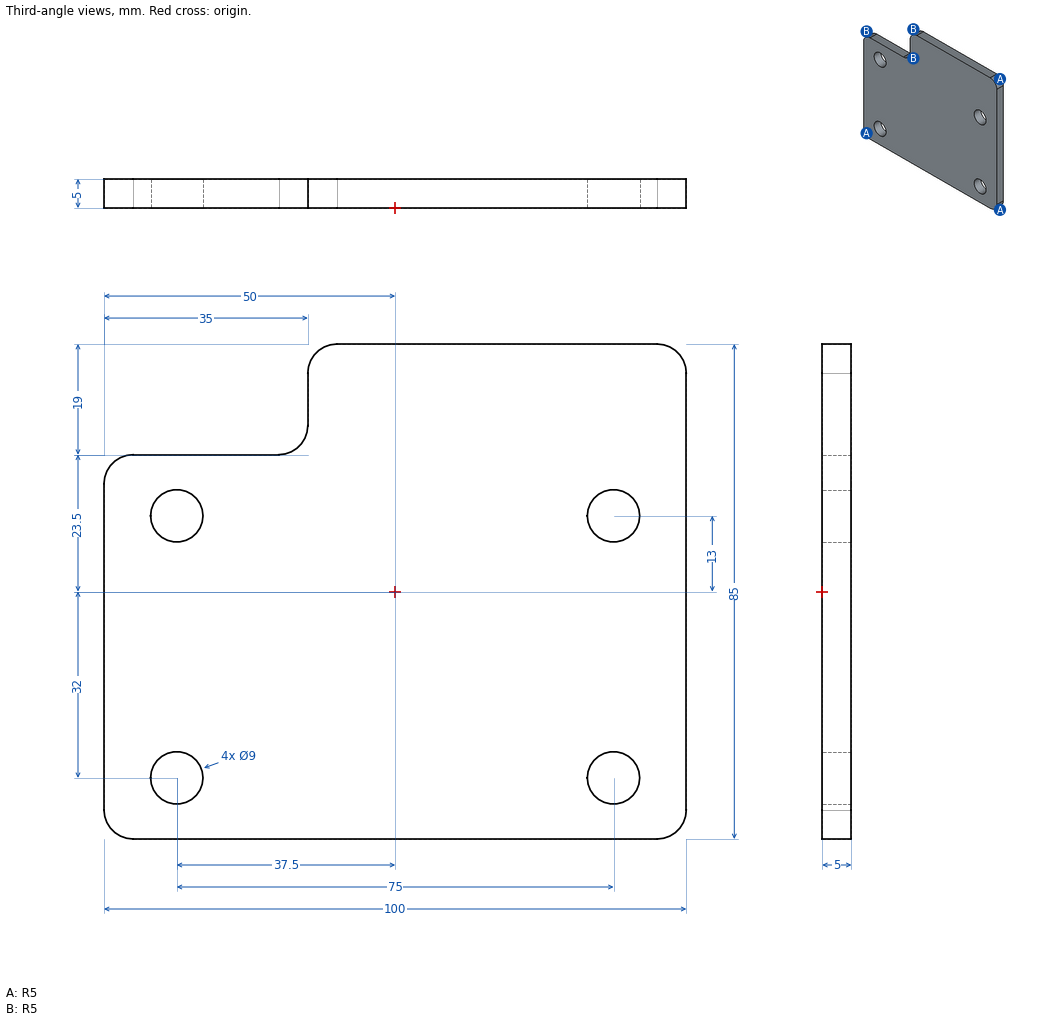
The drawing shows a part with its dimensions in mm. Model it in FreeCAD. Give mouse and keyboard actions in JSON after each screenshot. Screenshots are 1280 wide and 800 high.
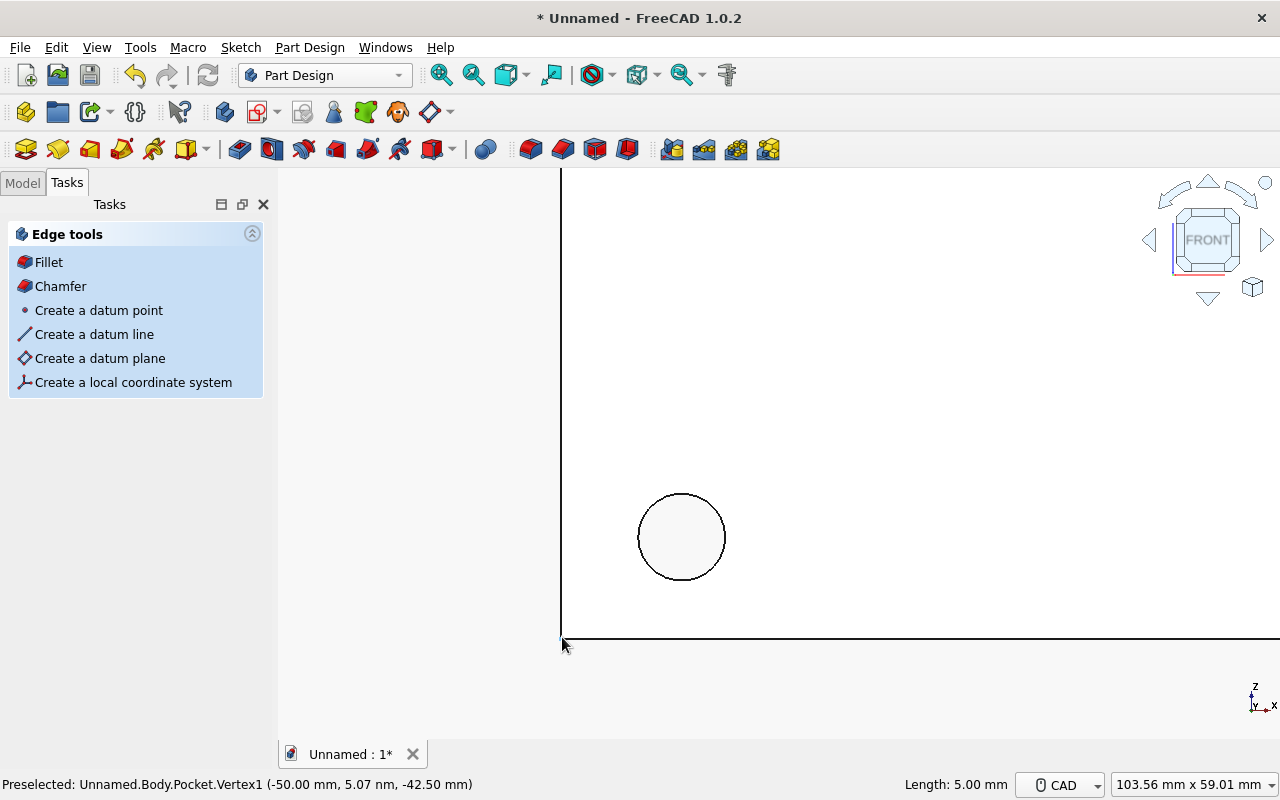
{"action": "left_click", "coordinate": [442, 76]}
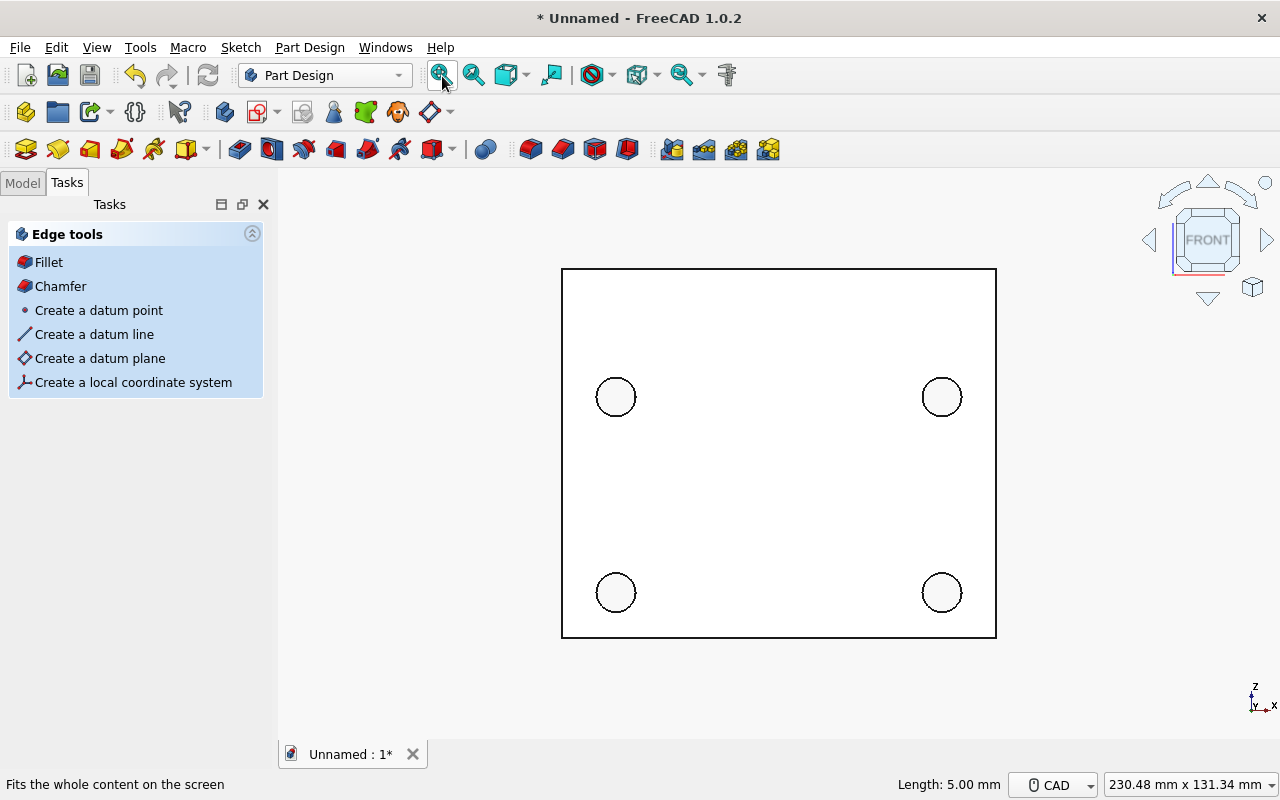
{"action": "key", "text": "3"}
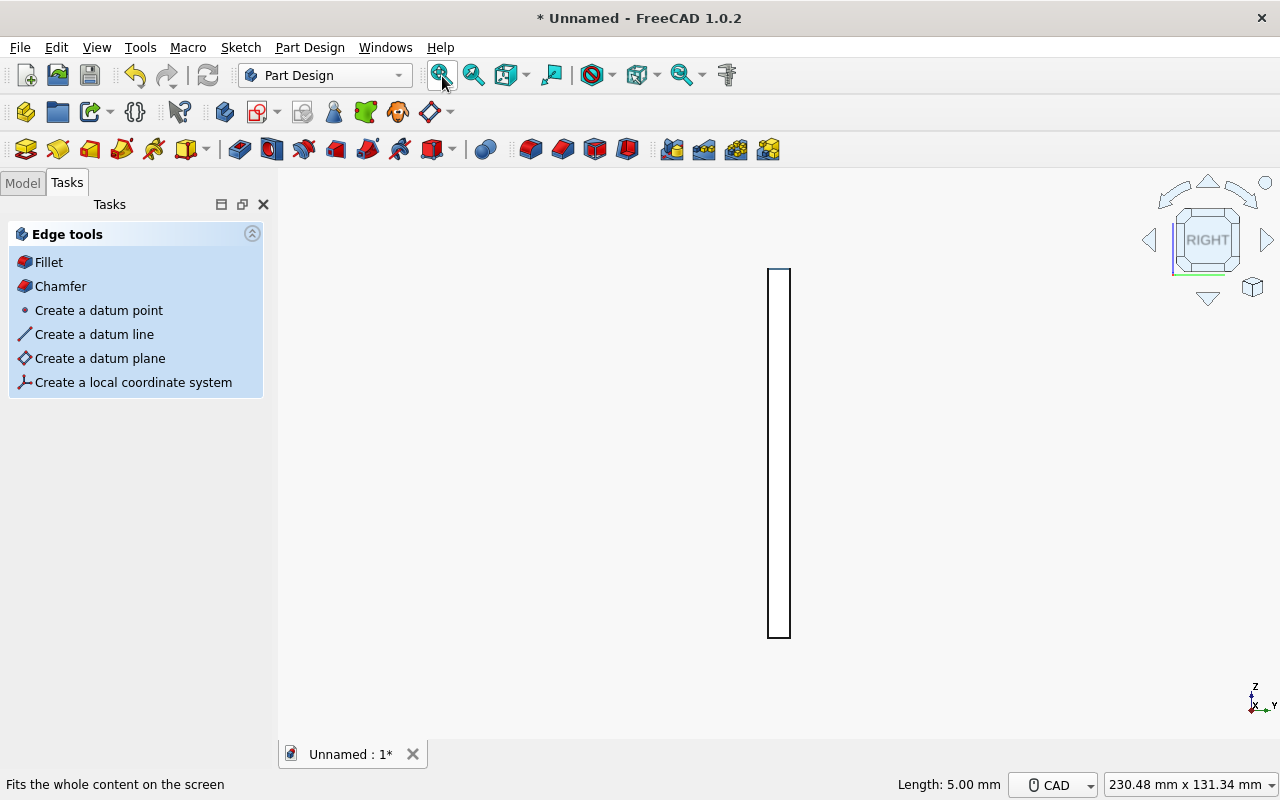
{"action": "left_click", "coordinate": [779, 637], "text": "ctrl"}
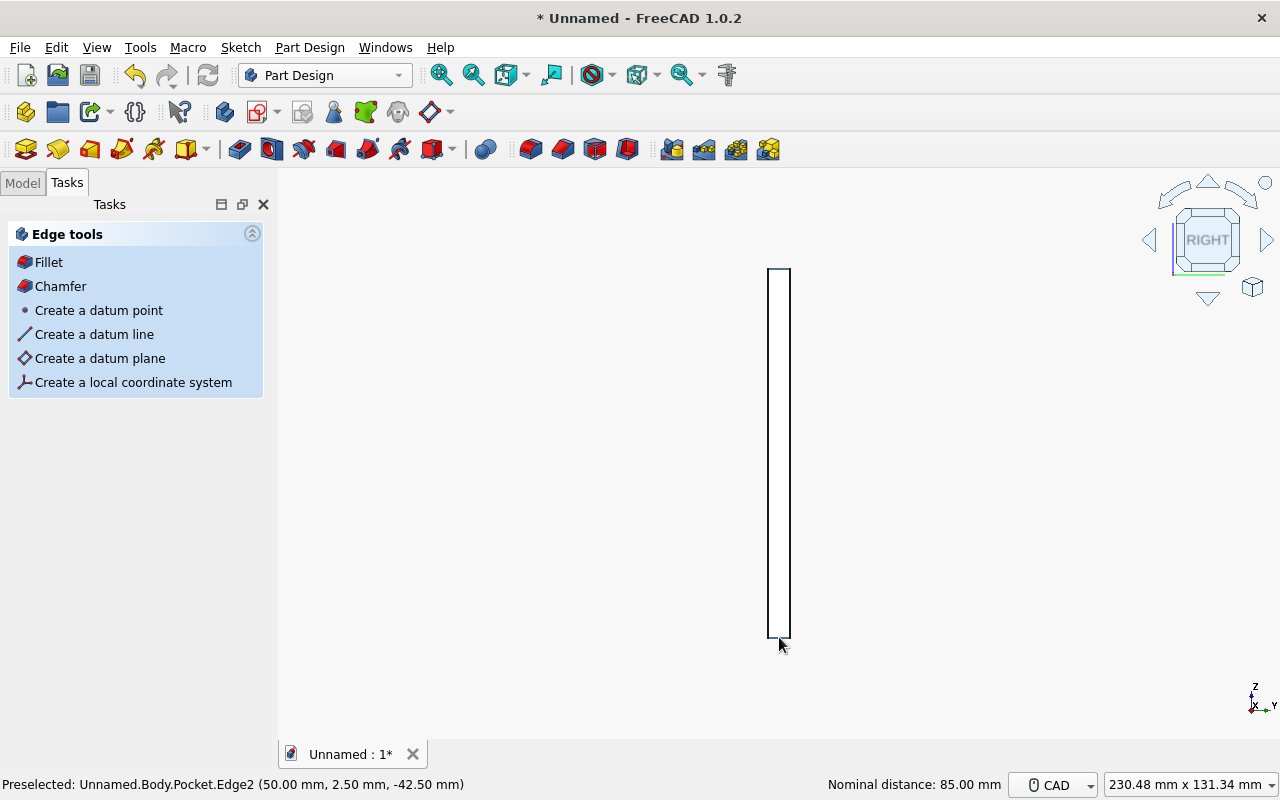
{"action": "scroll", "coordinate": [779, 637], "scroll_direction": "up", "scroll_amount": 4}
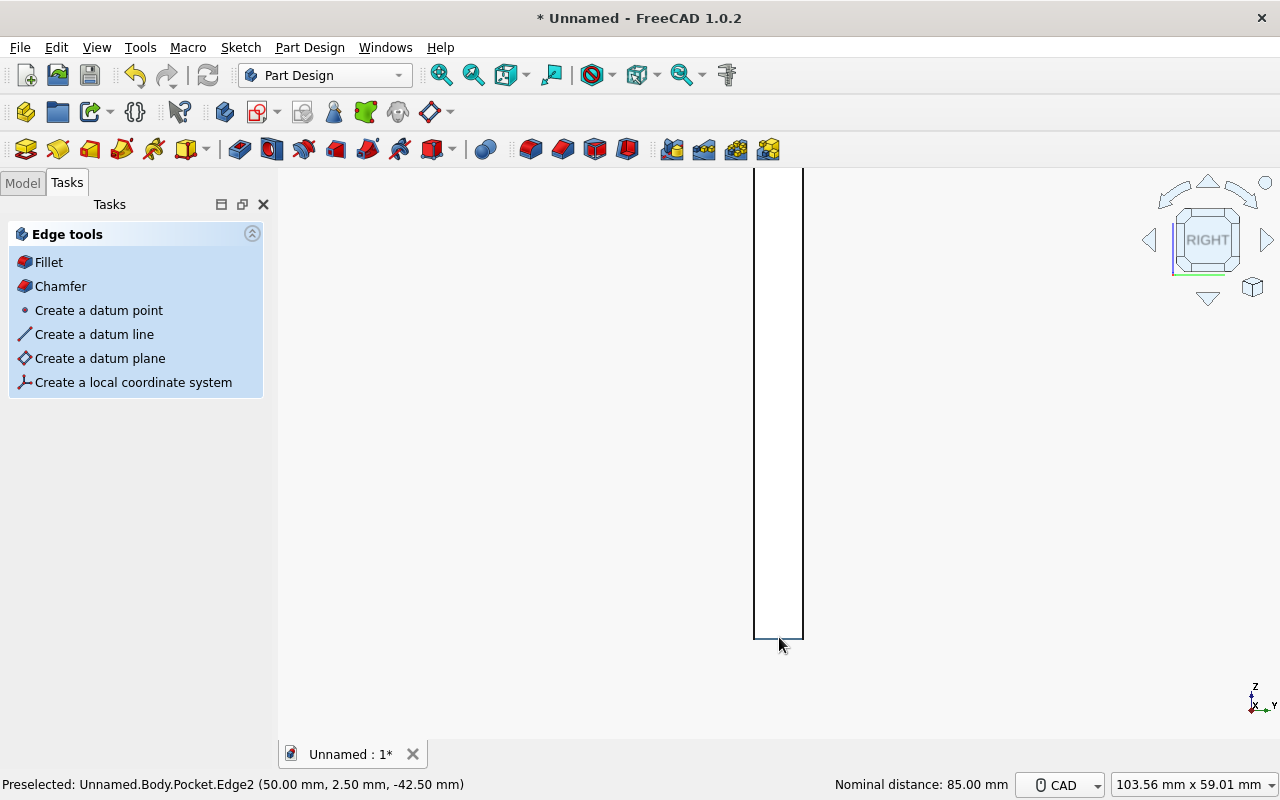
{"action": "left_click", "coordinate": [442, 76]}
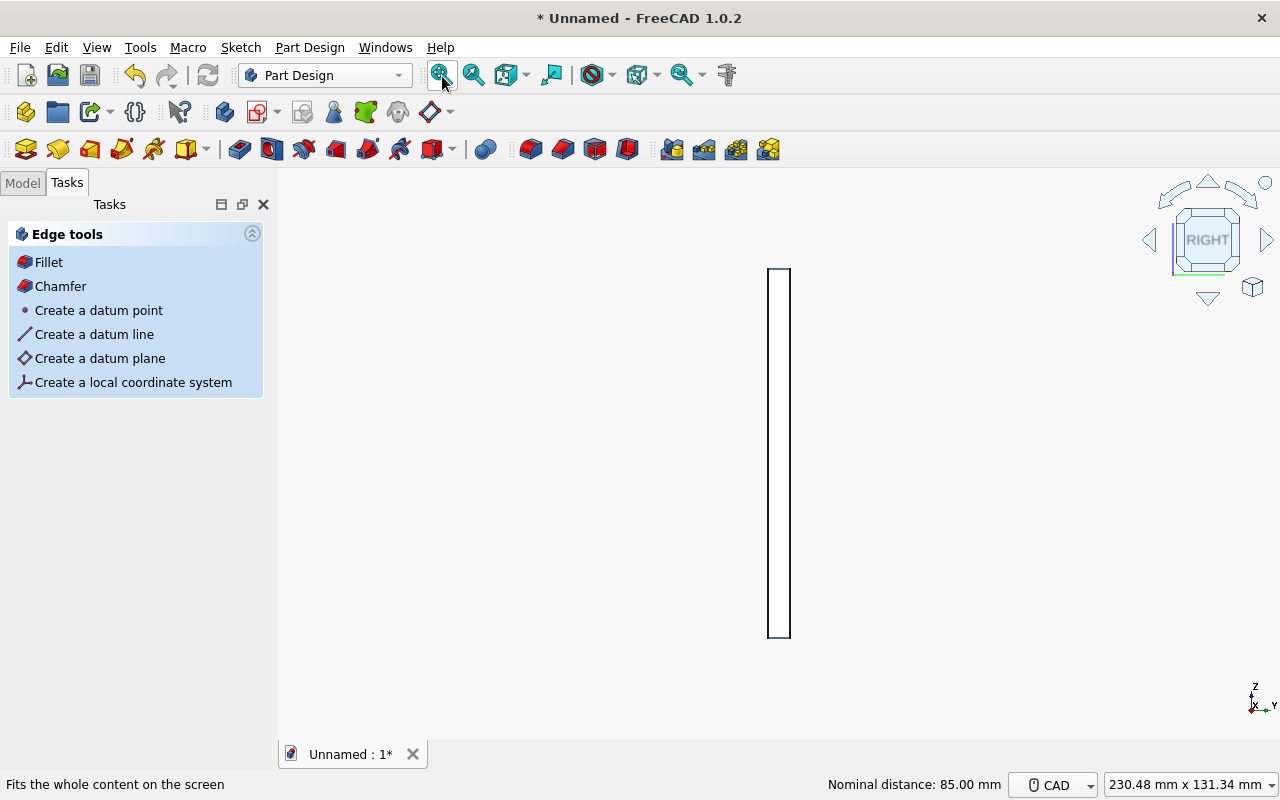
{"action": "key", "text": "5"}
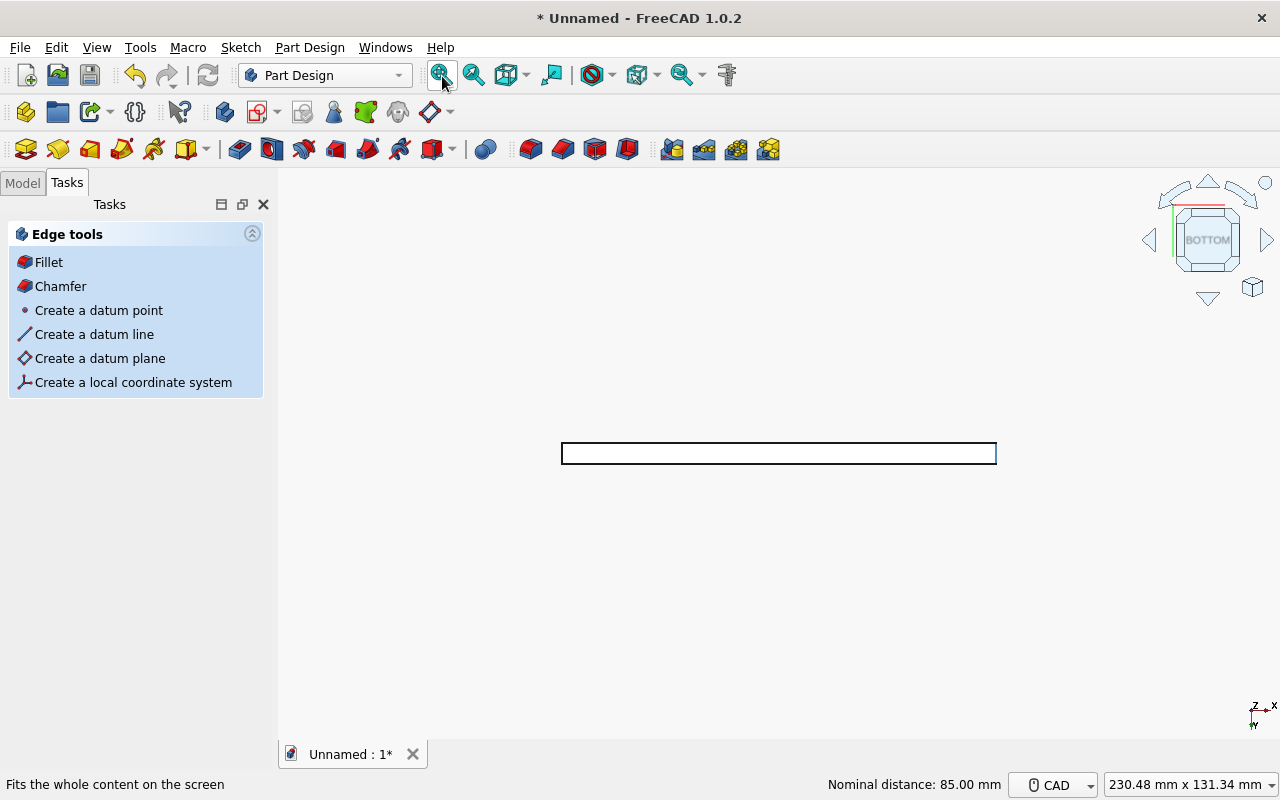
{"action": "left_click", "coordinate": [442, 76]}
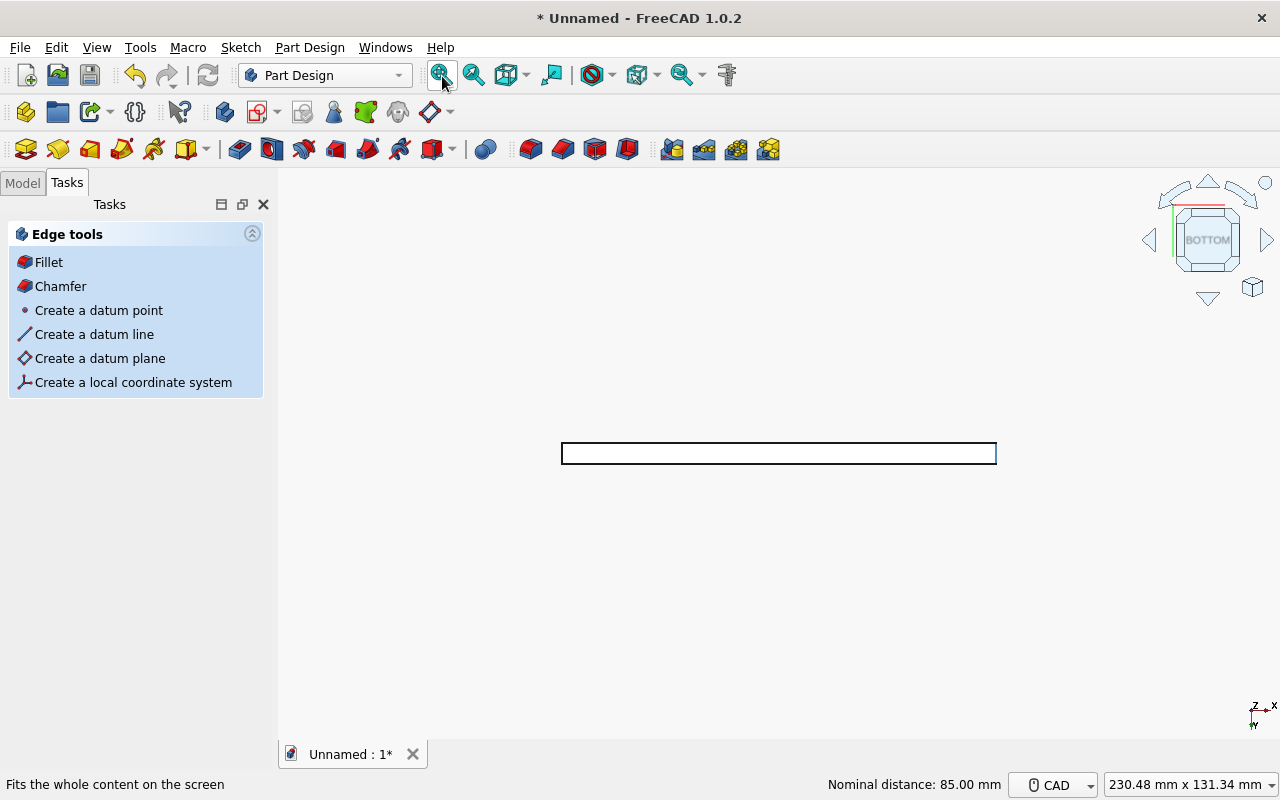
{"action": "left_click", "coordinate": [562, 452], "text": "ctrl"}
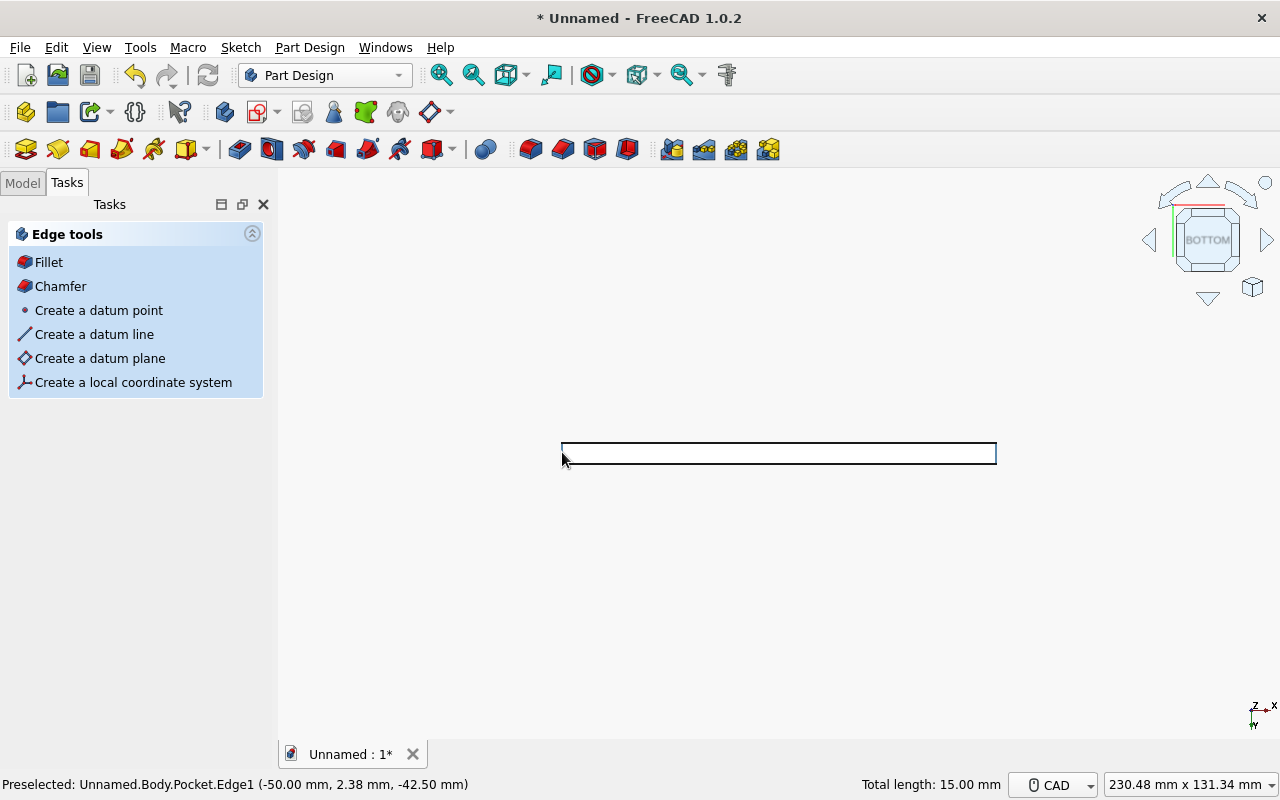
{"action": "left_click", "coordinate": [532, 150]}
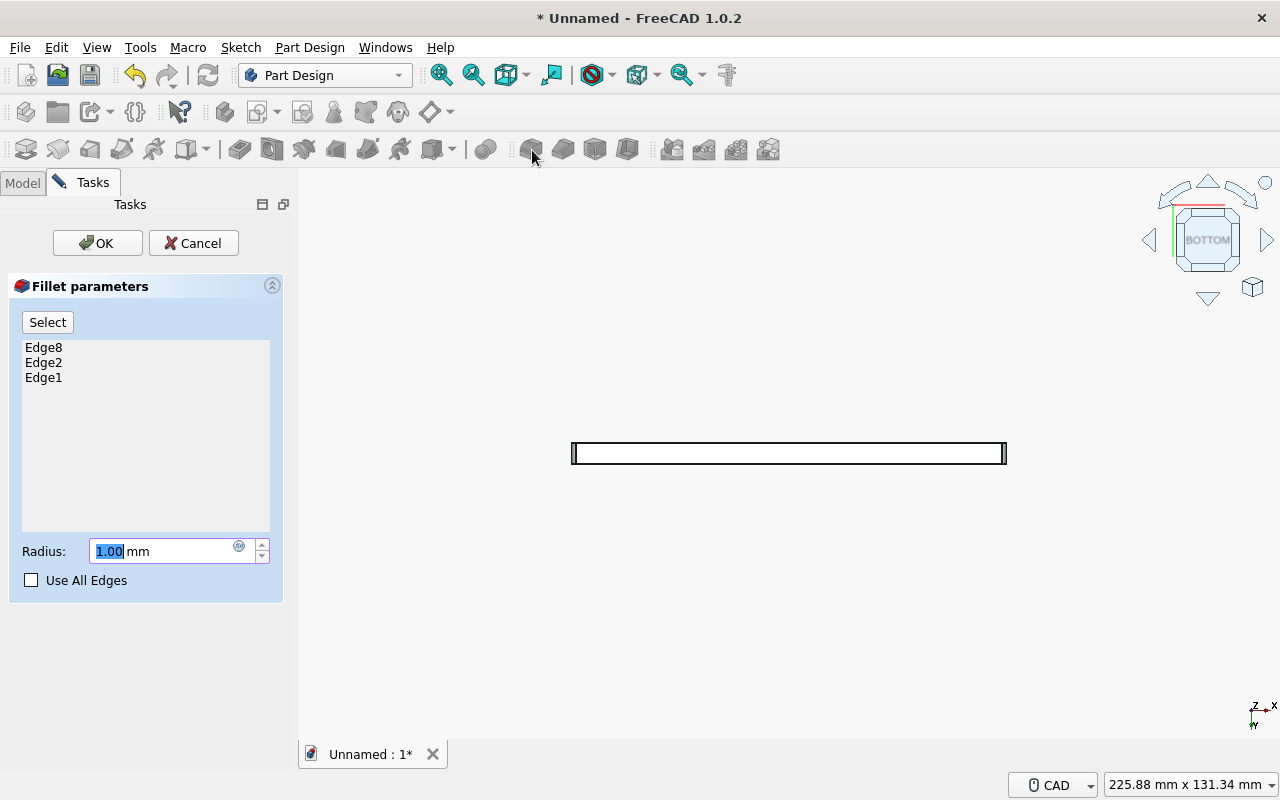
{"action": "type", "text": "5"}
{"action": "key", "text": "Tab"}